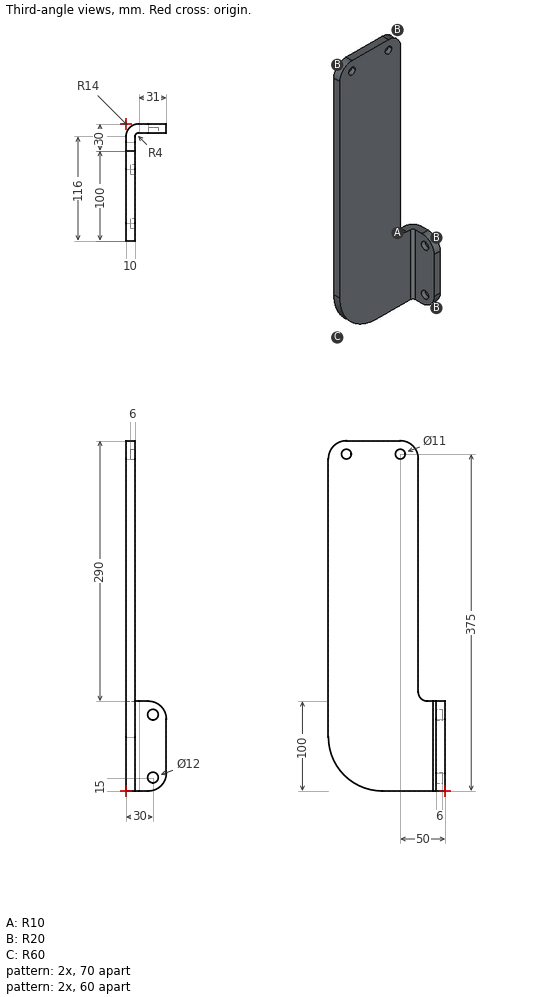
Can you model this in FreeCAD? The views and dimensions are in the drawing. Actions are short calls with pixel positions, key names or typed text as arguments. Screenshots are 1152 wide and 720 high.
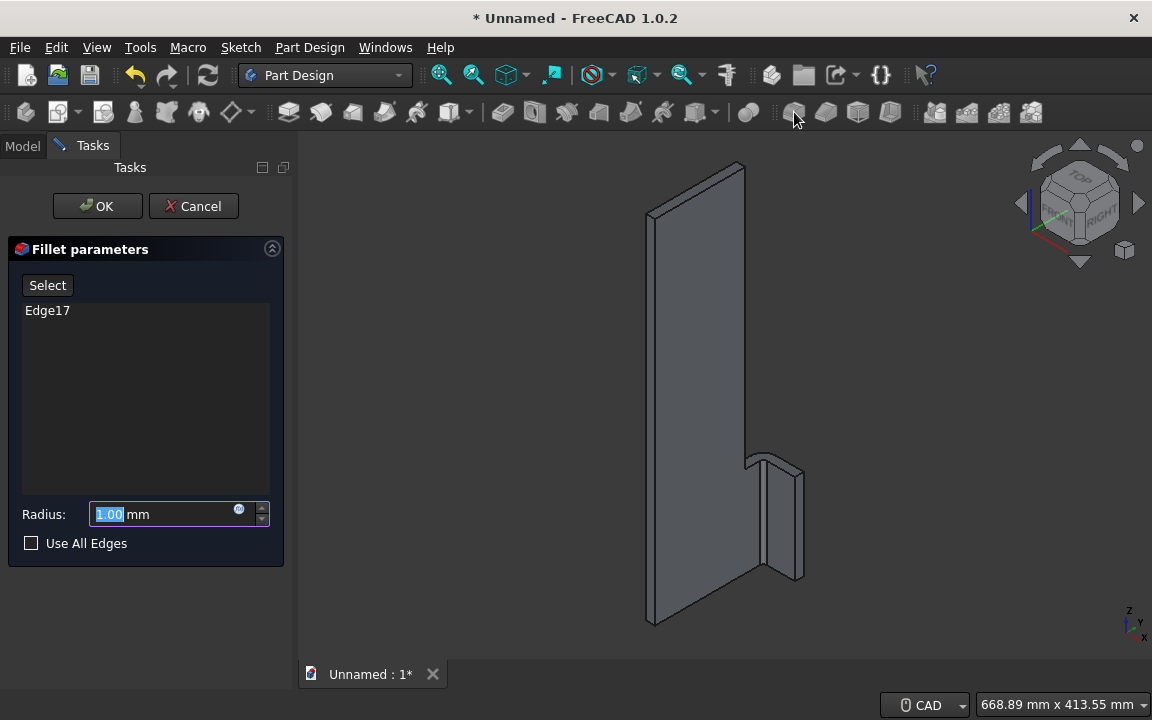
text(10)
key(Tab)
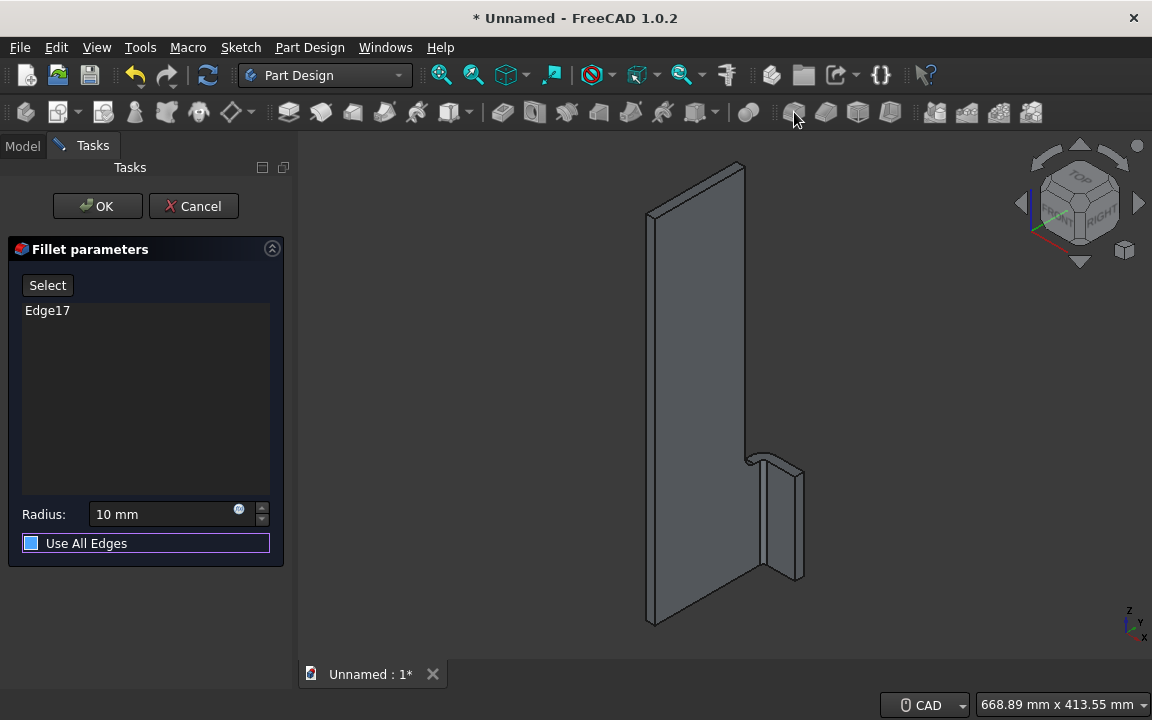
click(98, 206)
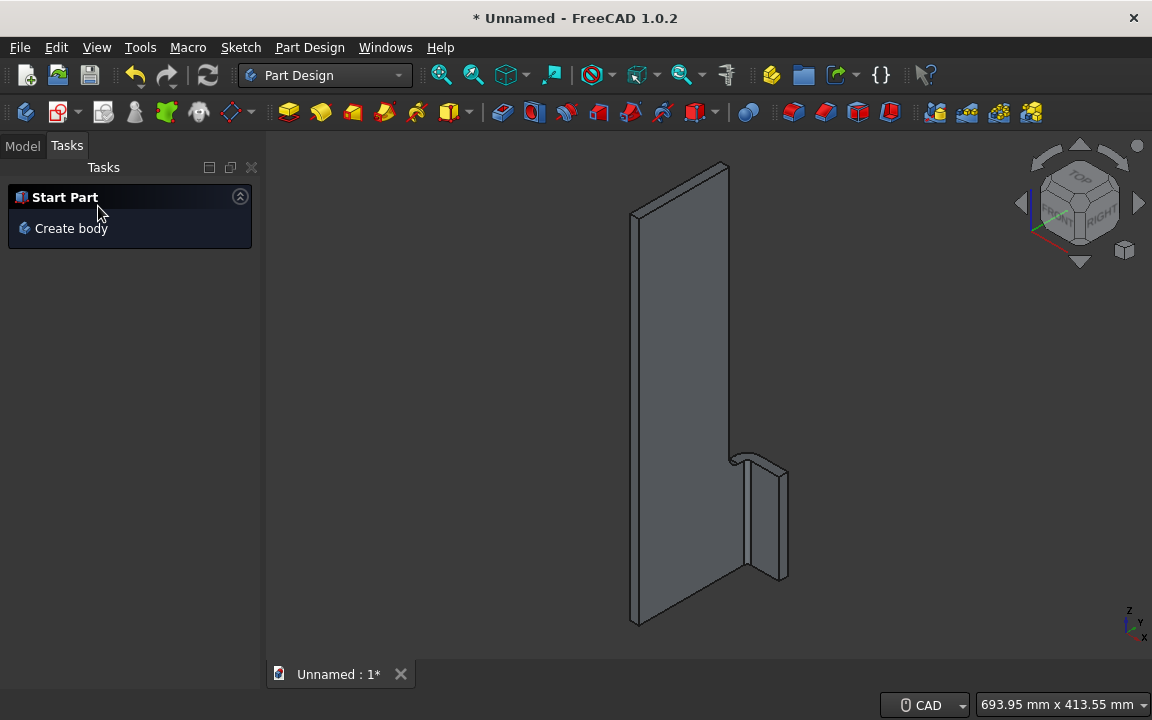
click(633, 214)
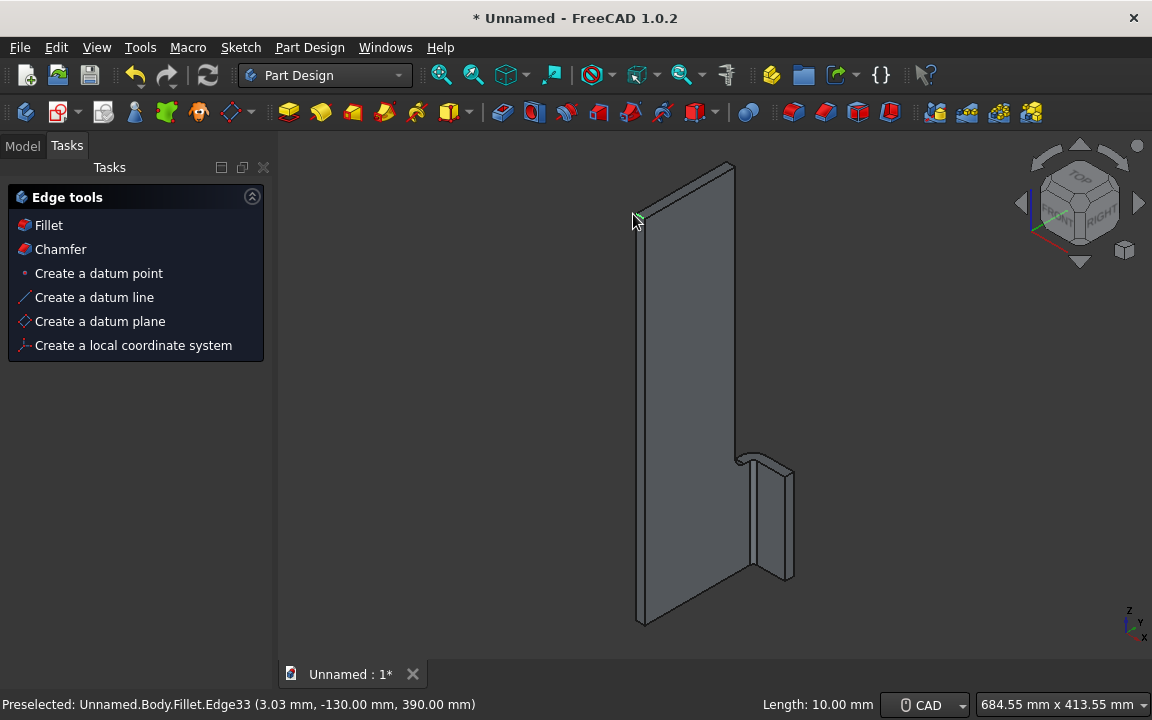
click(791, 472, ctrl)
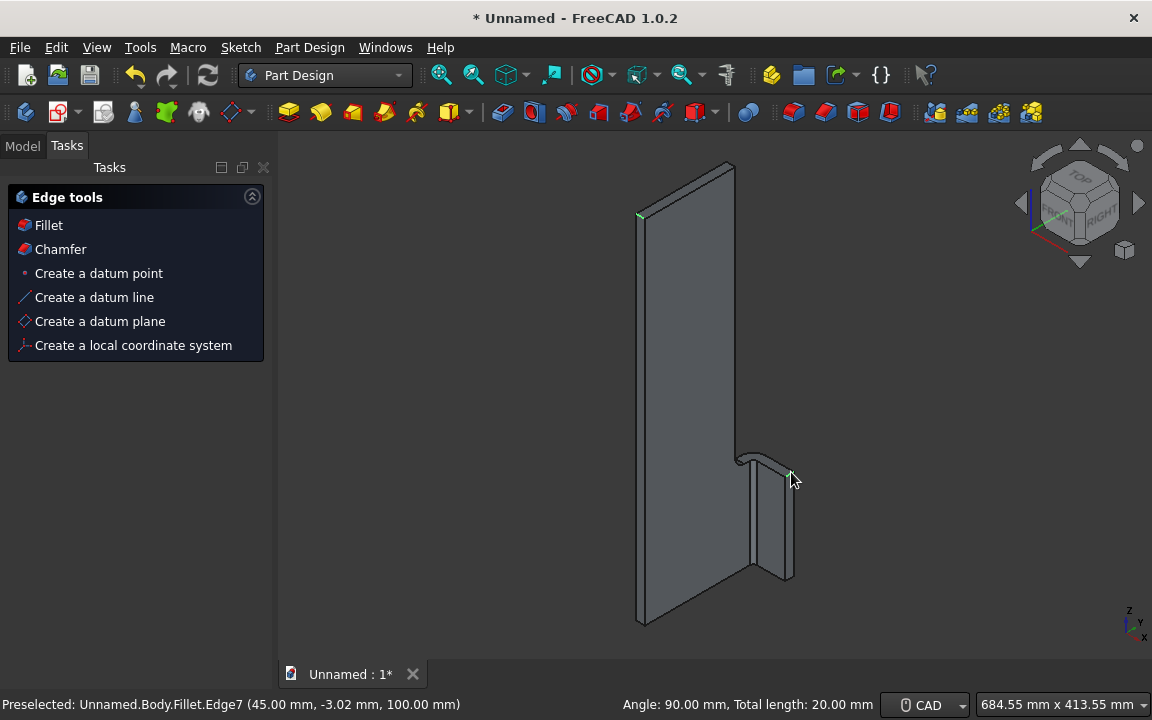
scroll(731, 163, up, 6)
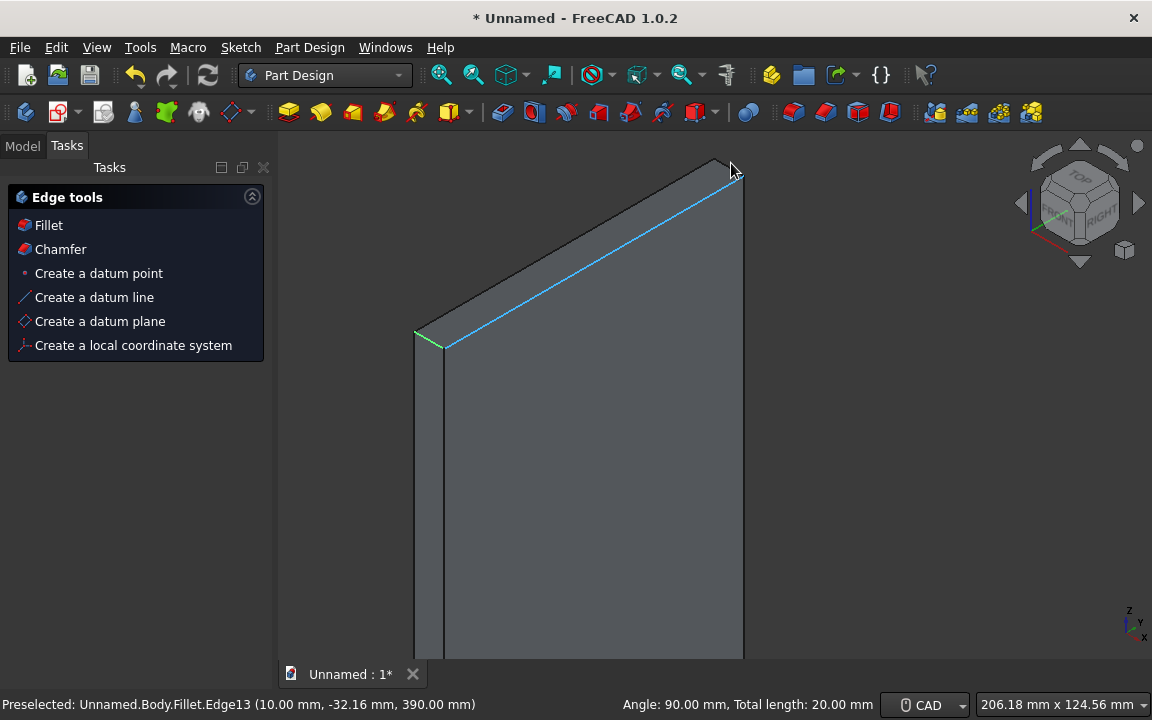
click(442, 76)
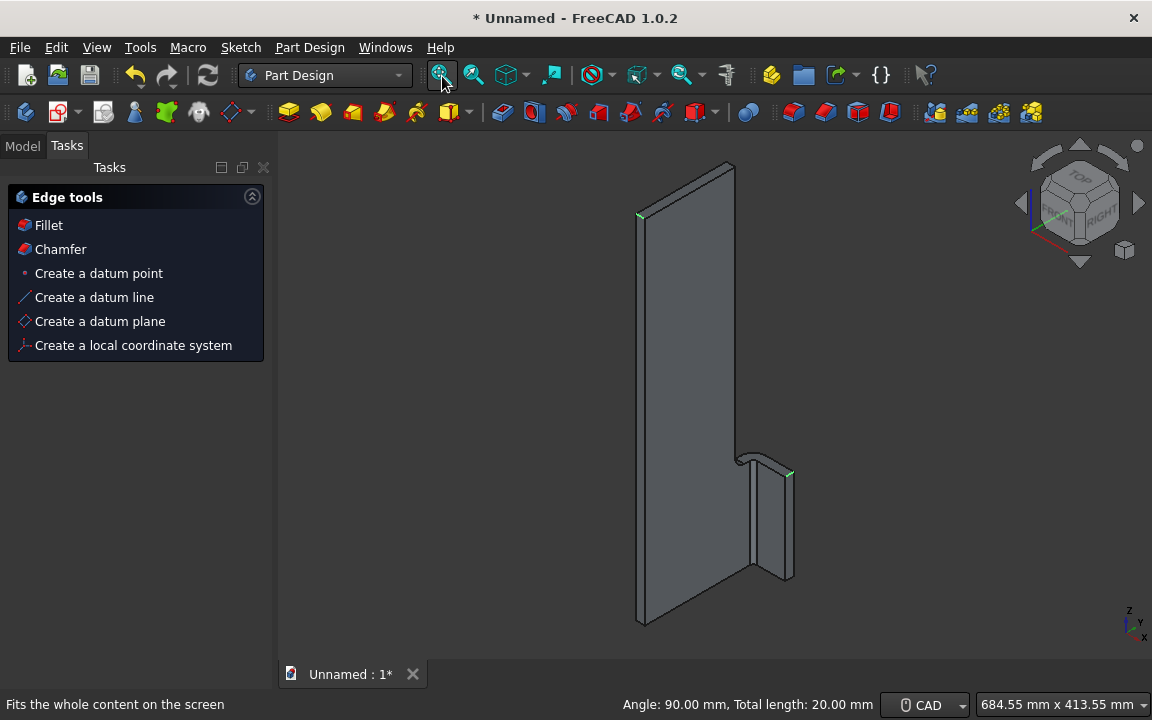
key(2)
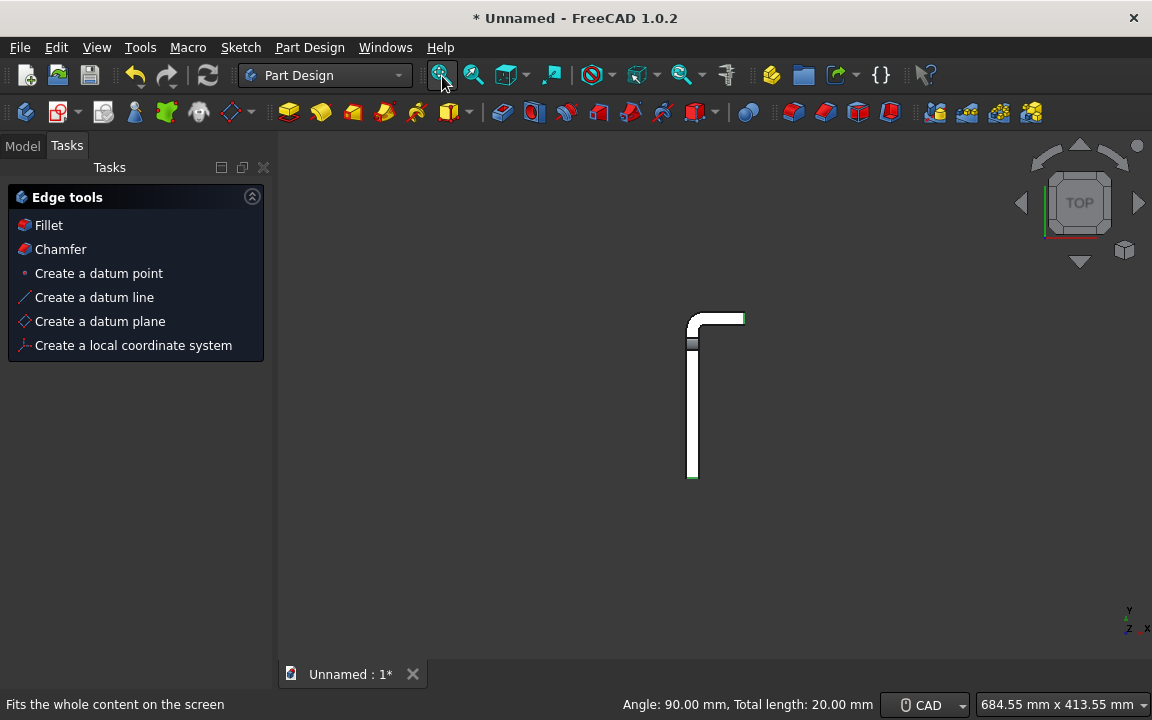
click(442, 76)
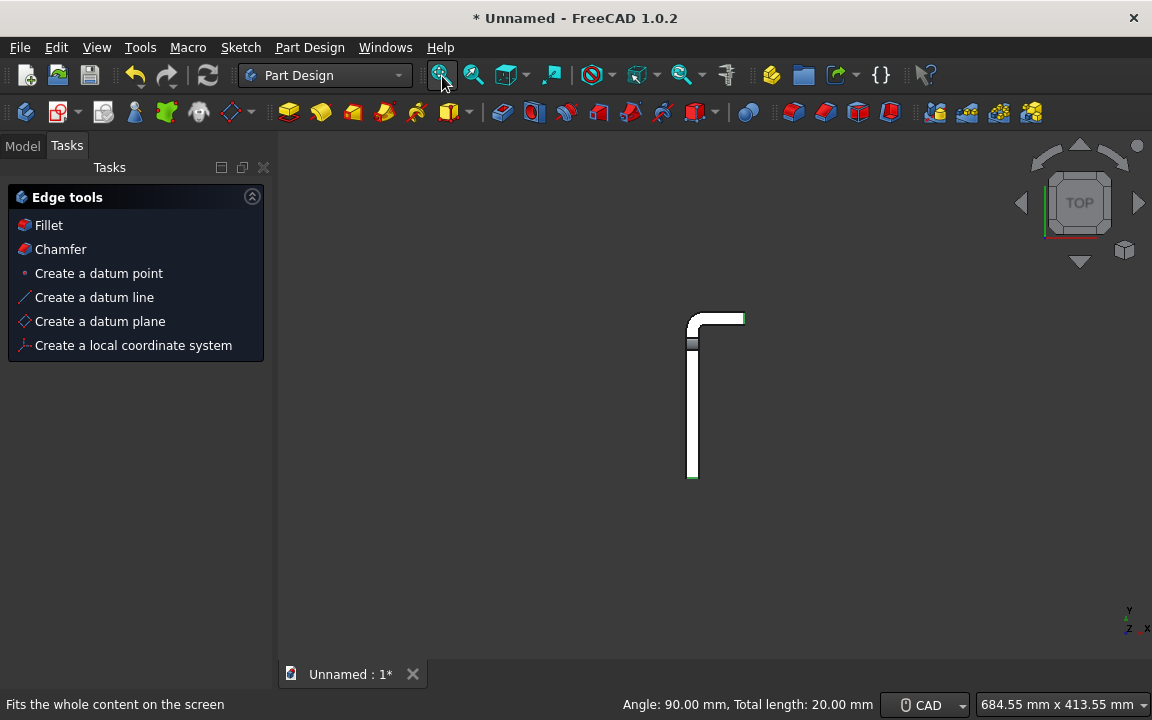
click(693, 349, ctrl)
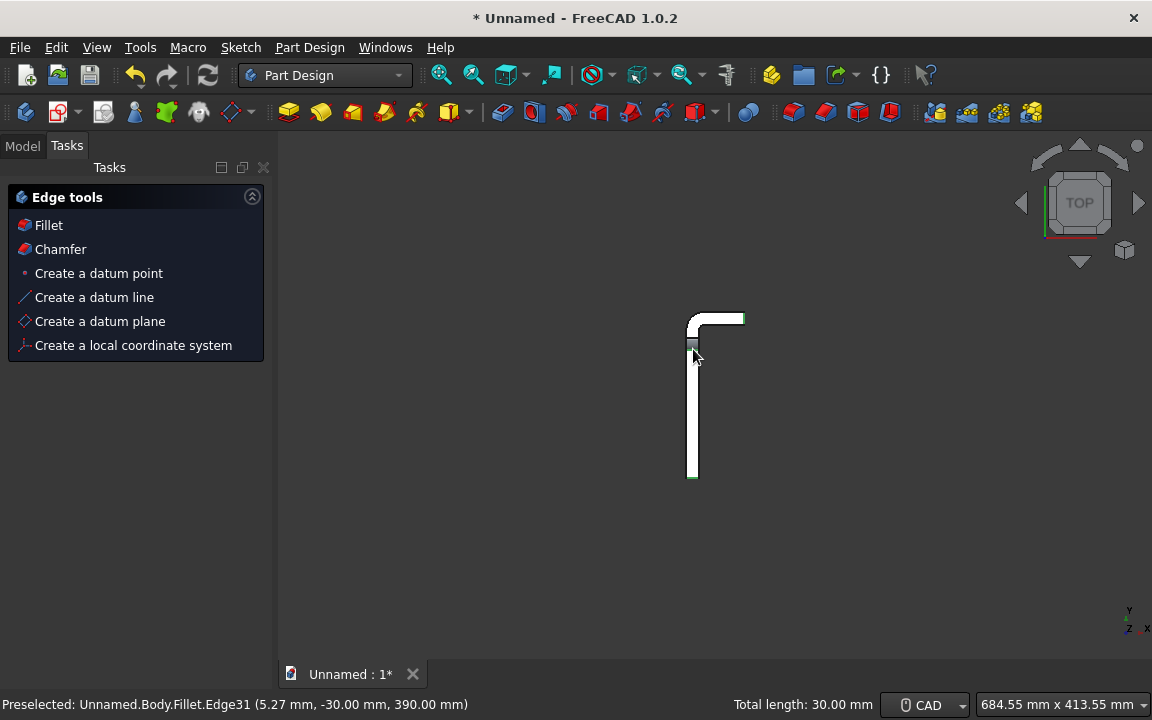
scroll(744, 317, up, 6)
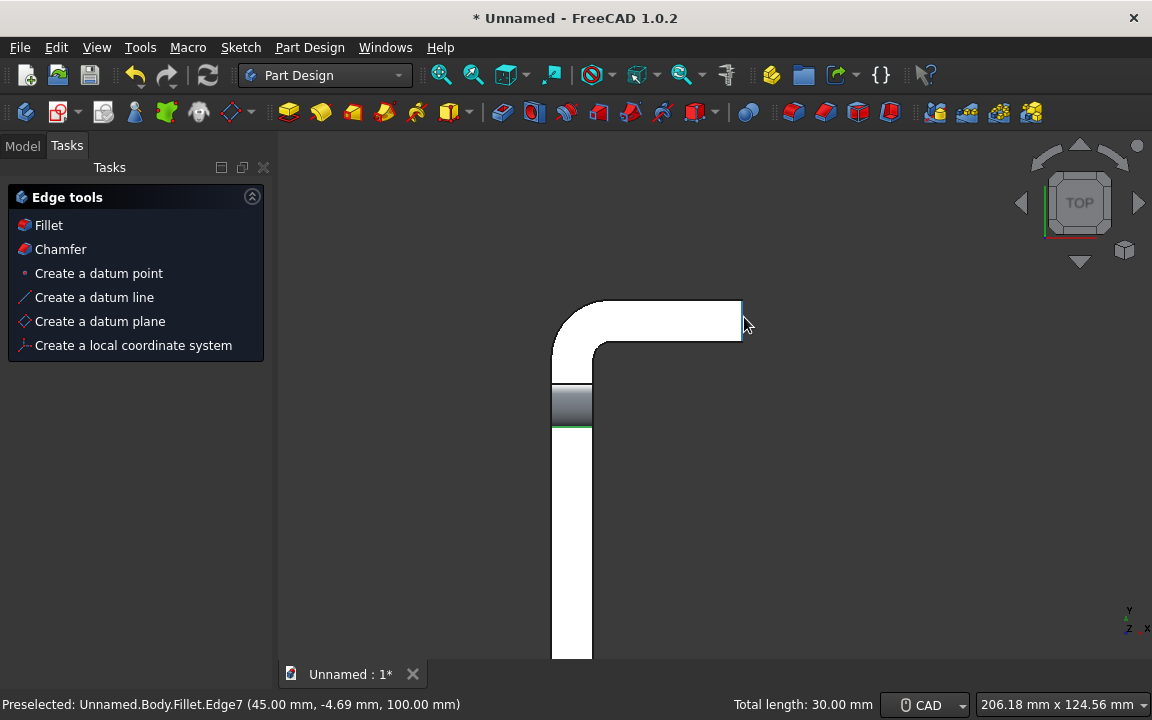
click(442, 76)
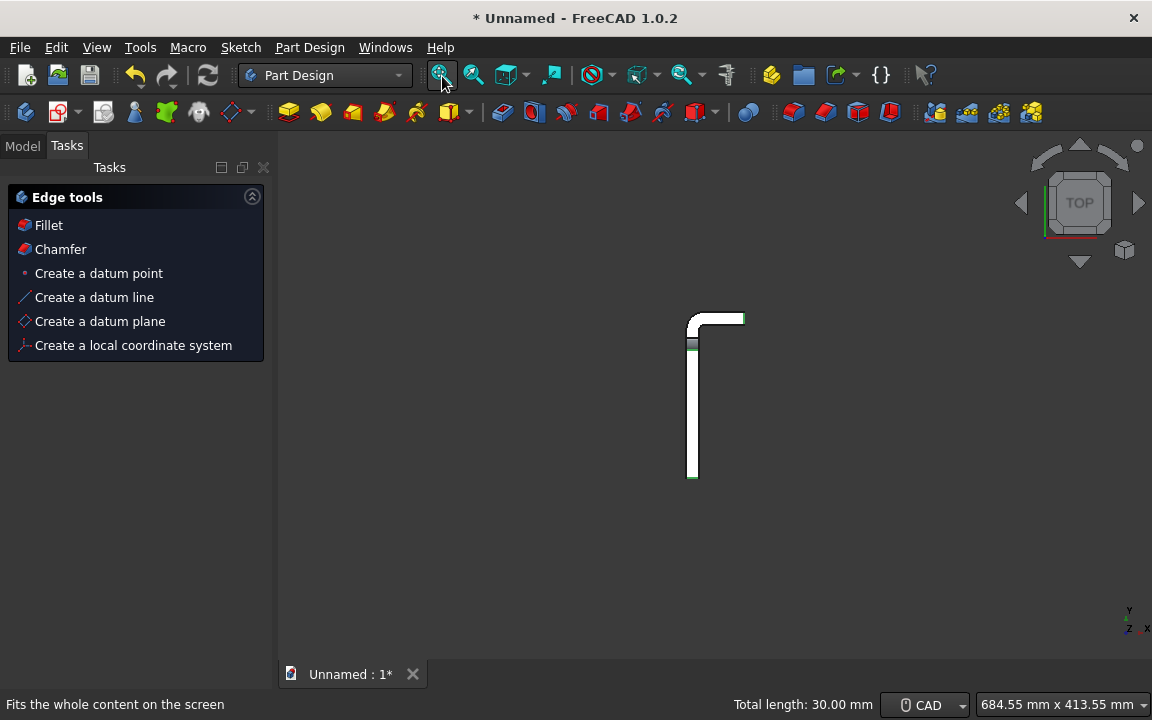
key(0)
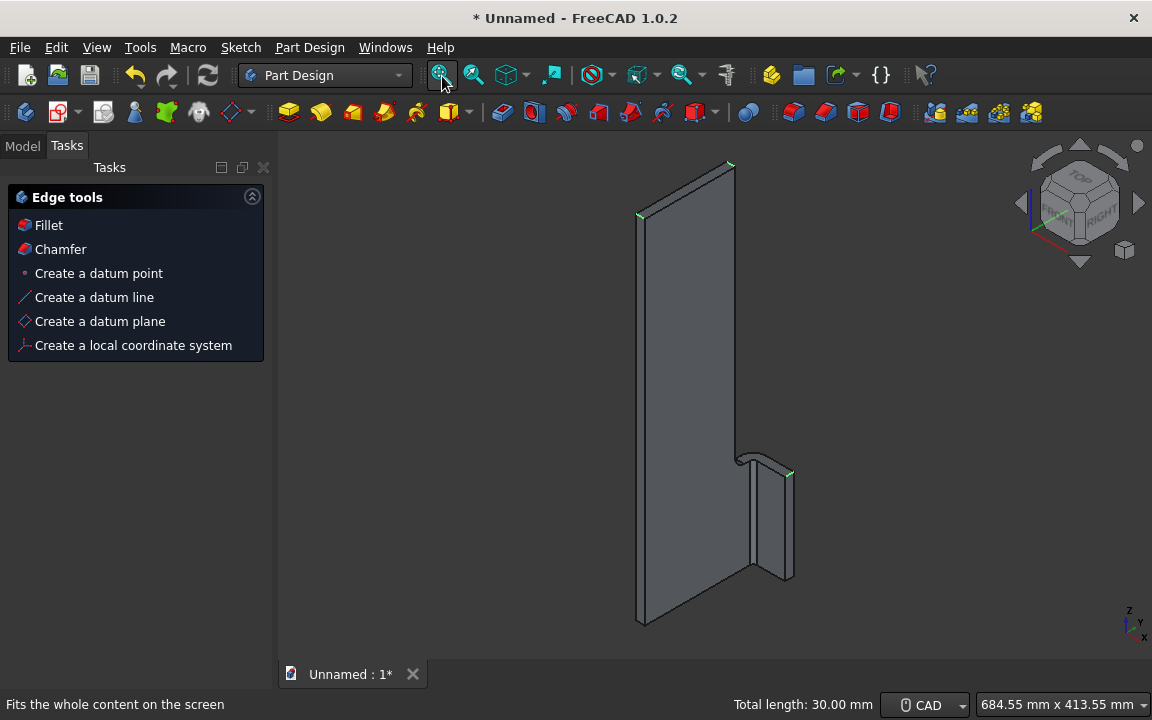
scroll(789, 578, up, 6)